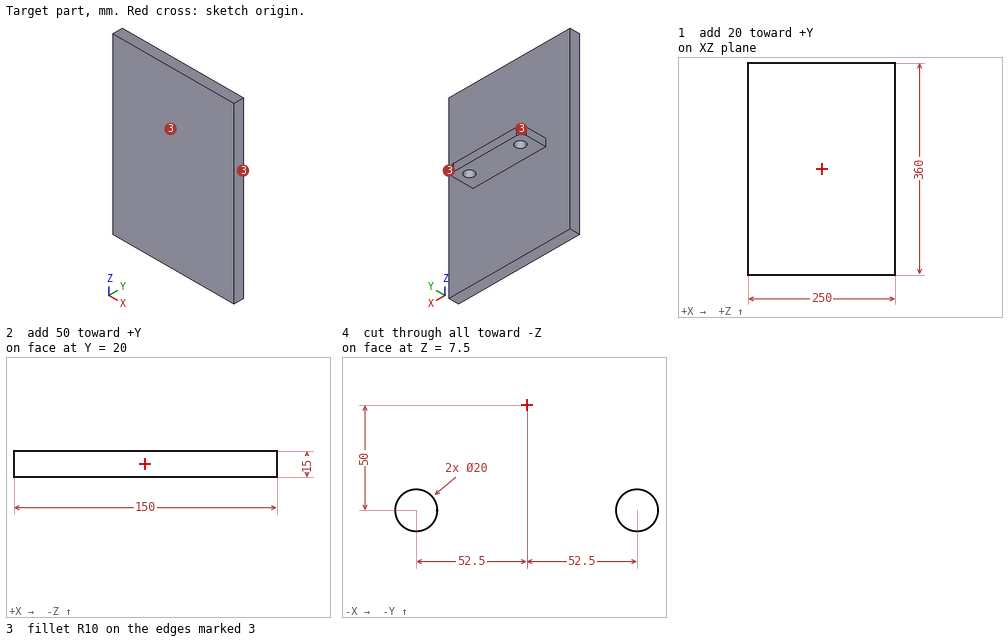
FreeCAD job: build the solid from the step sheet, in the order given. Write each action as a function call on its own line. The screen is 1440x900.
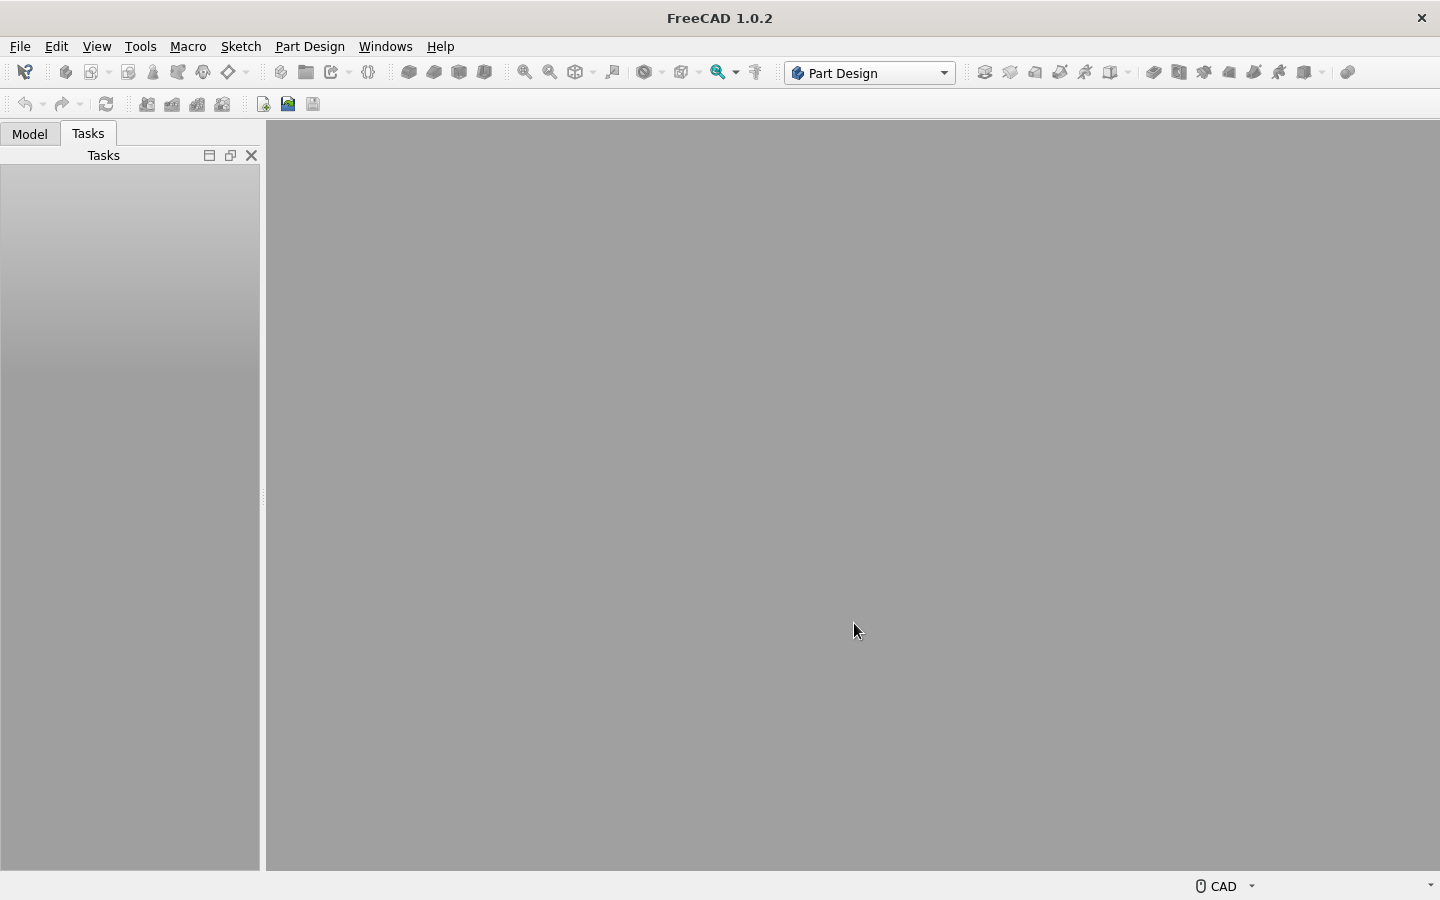
click(263, 104)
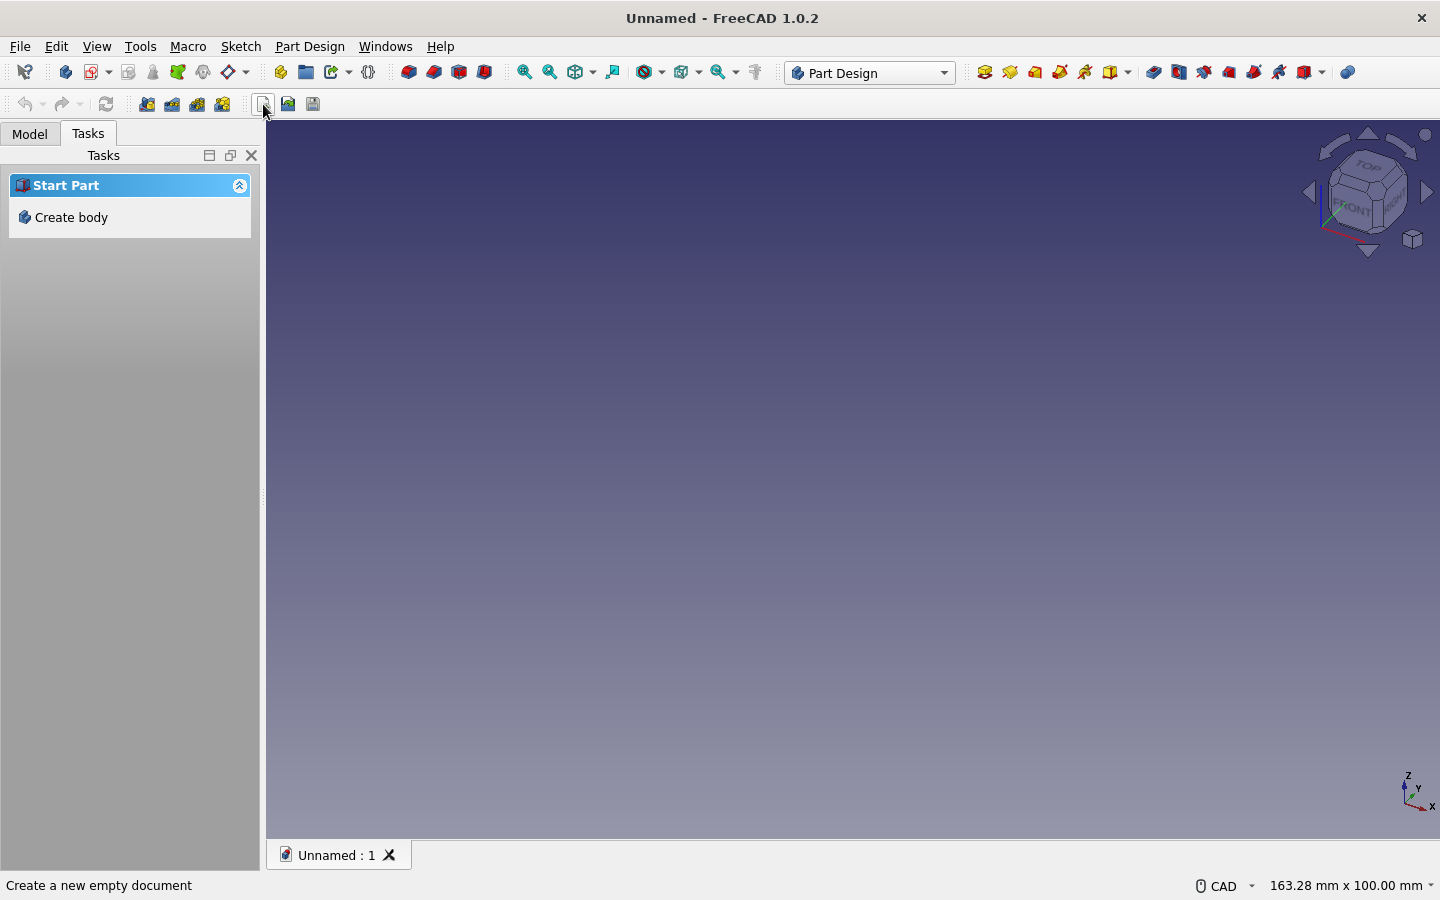
click(90, 72)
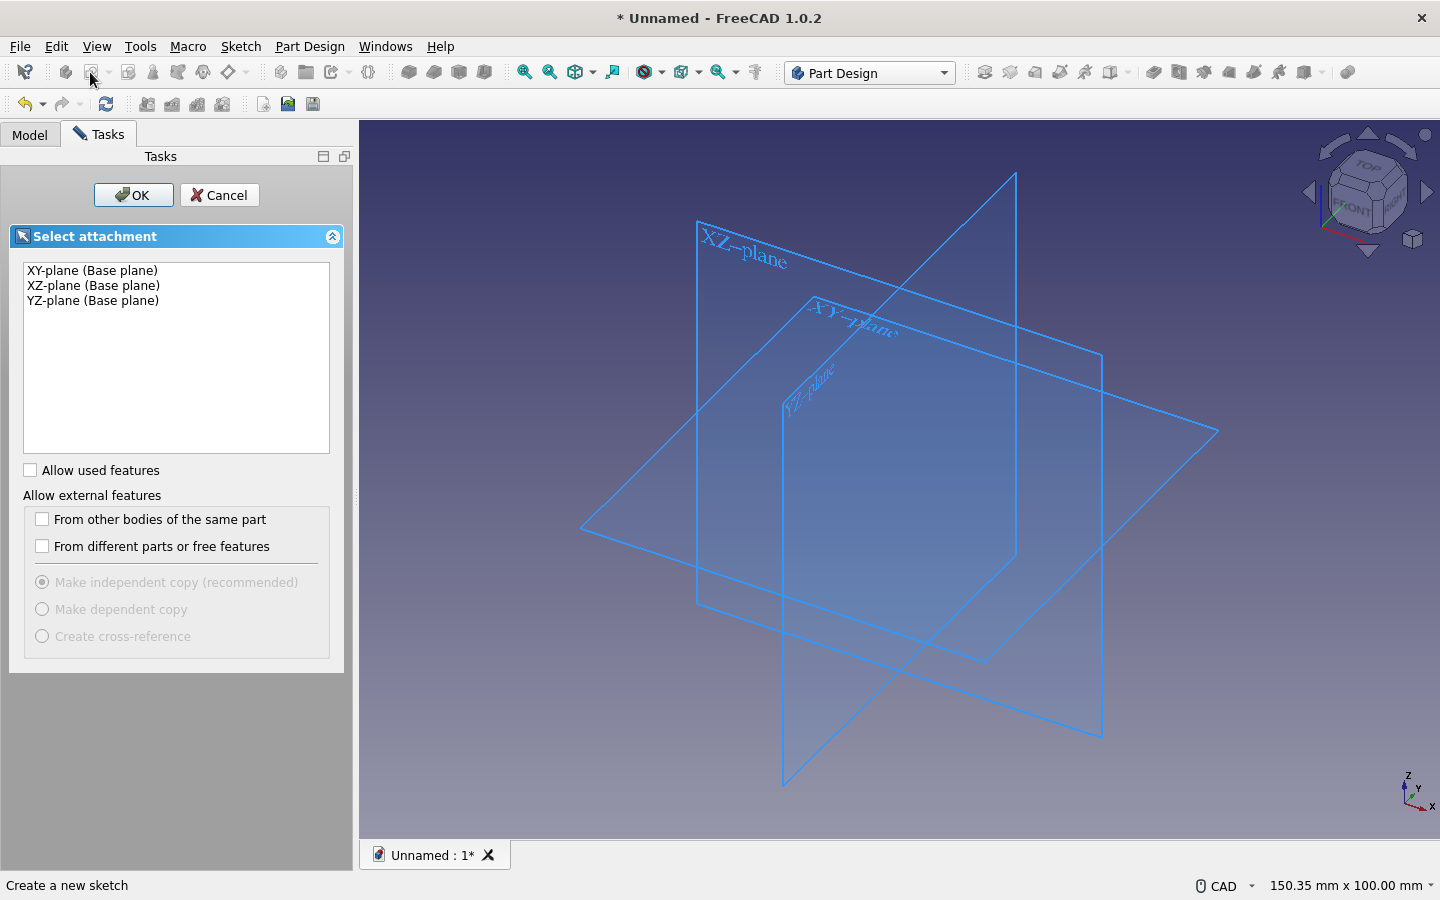
click(84, 286)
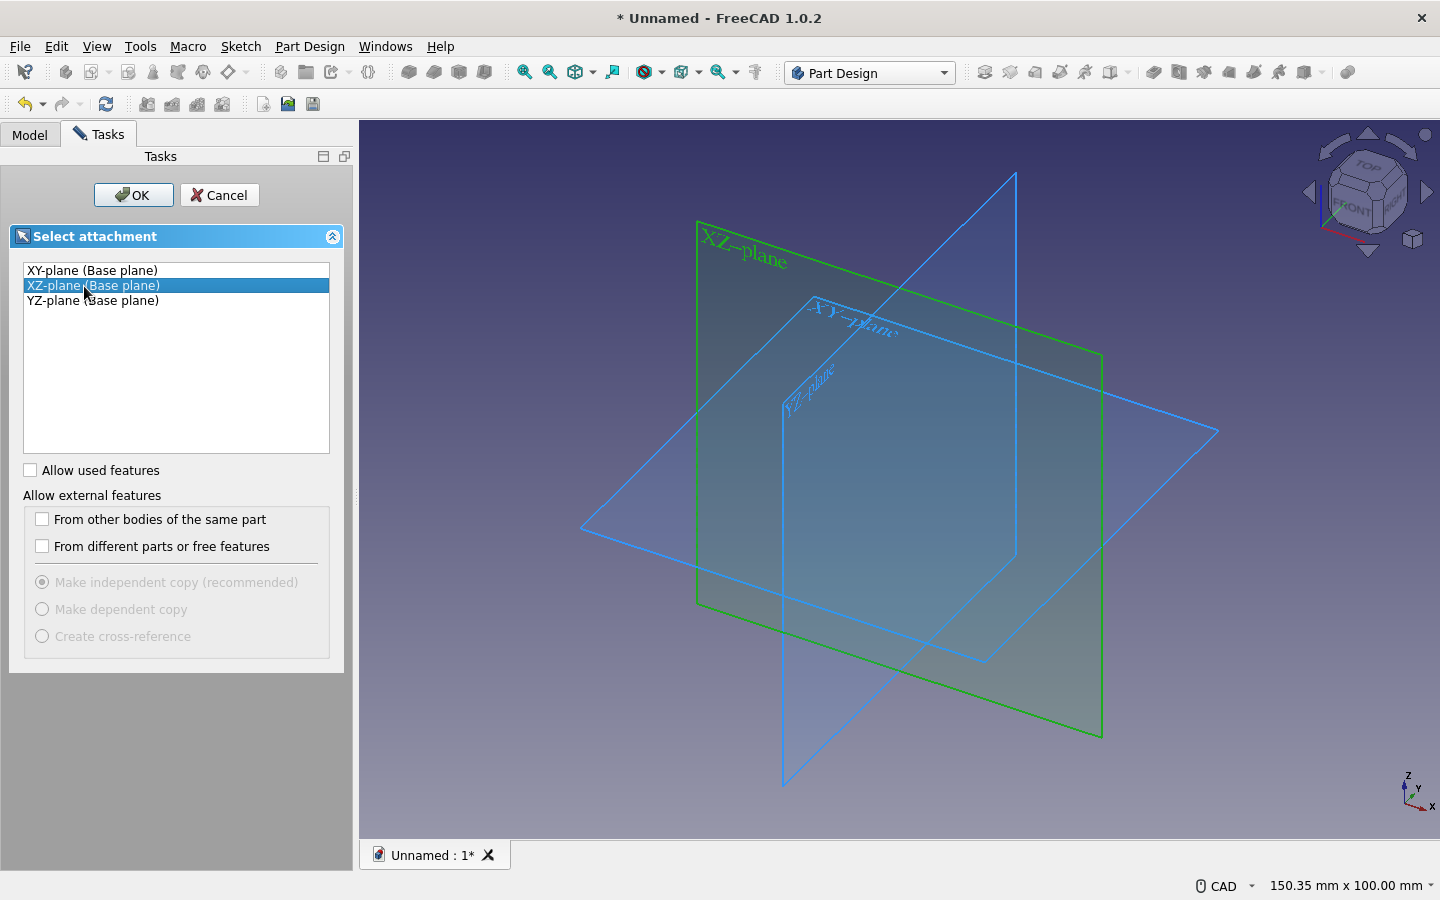
click(134, 195)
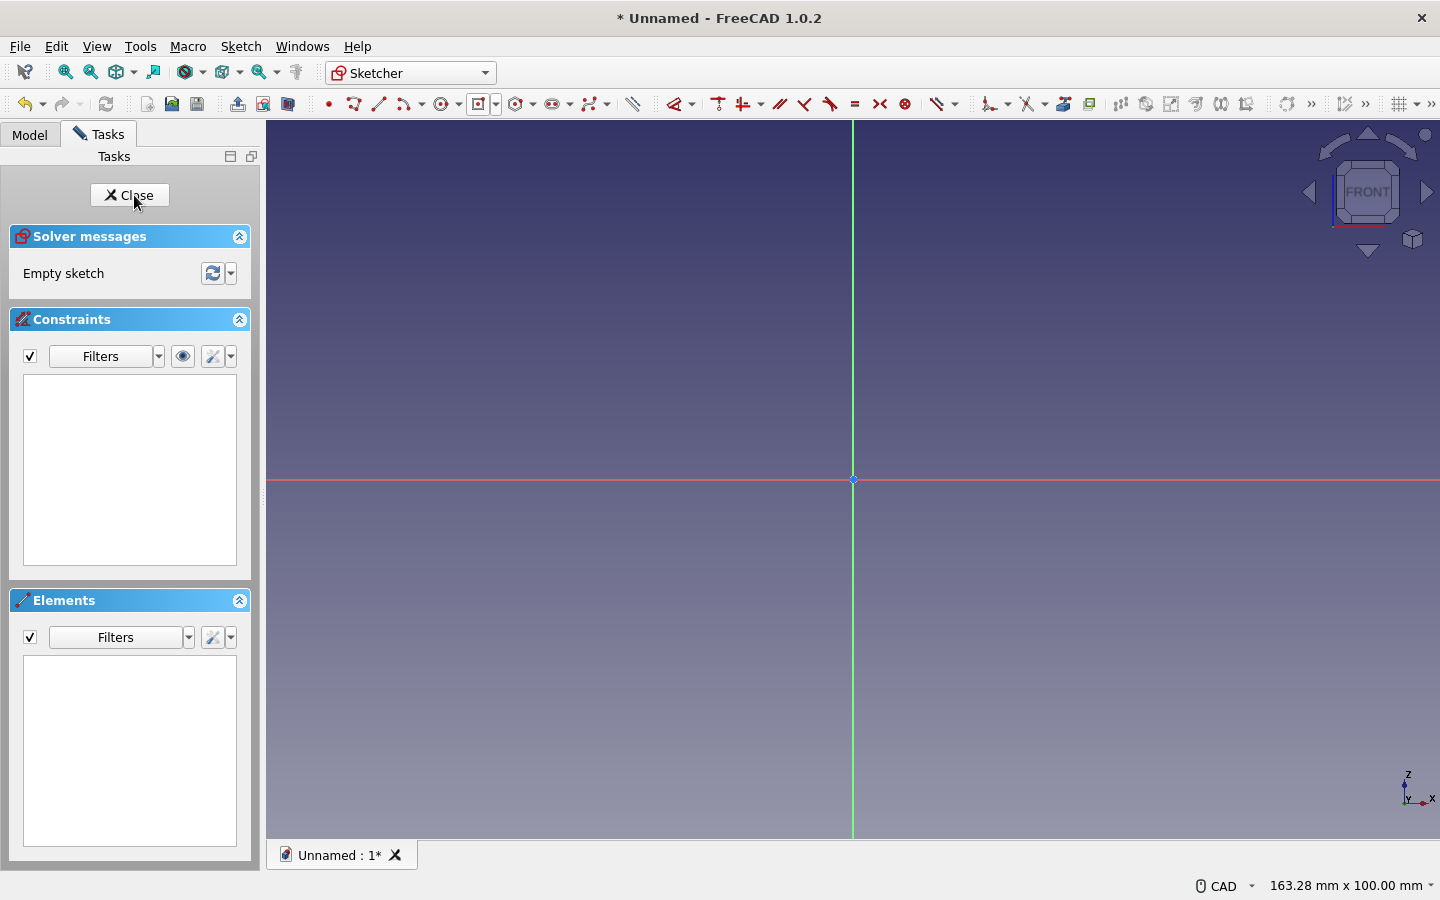
scroll(771, 480, down, 9)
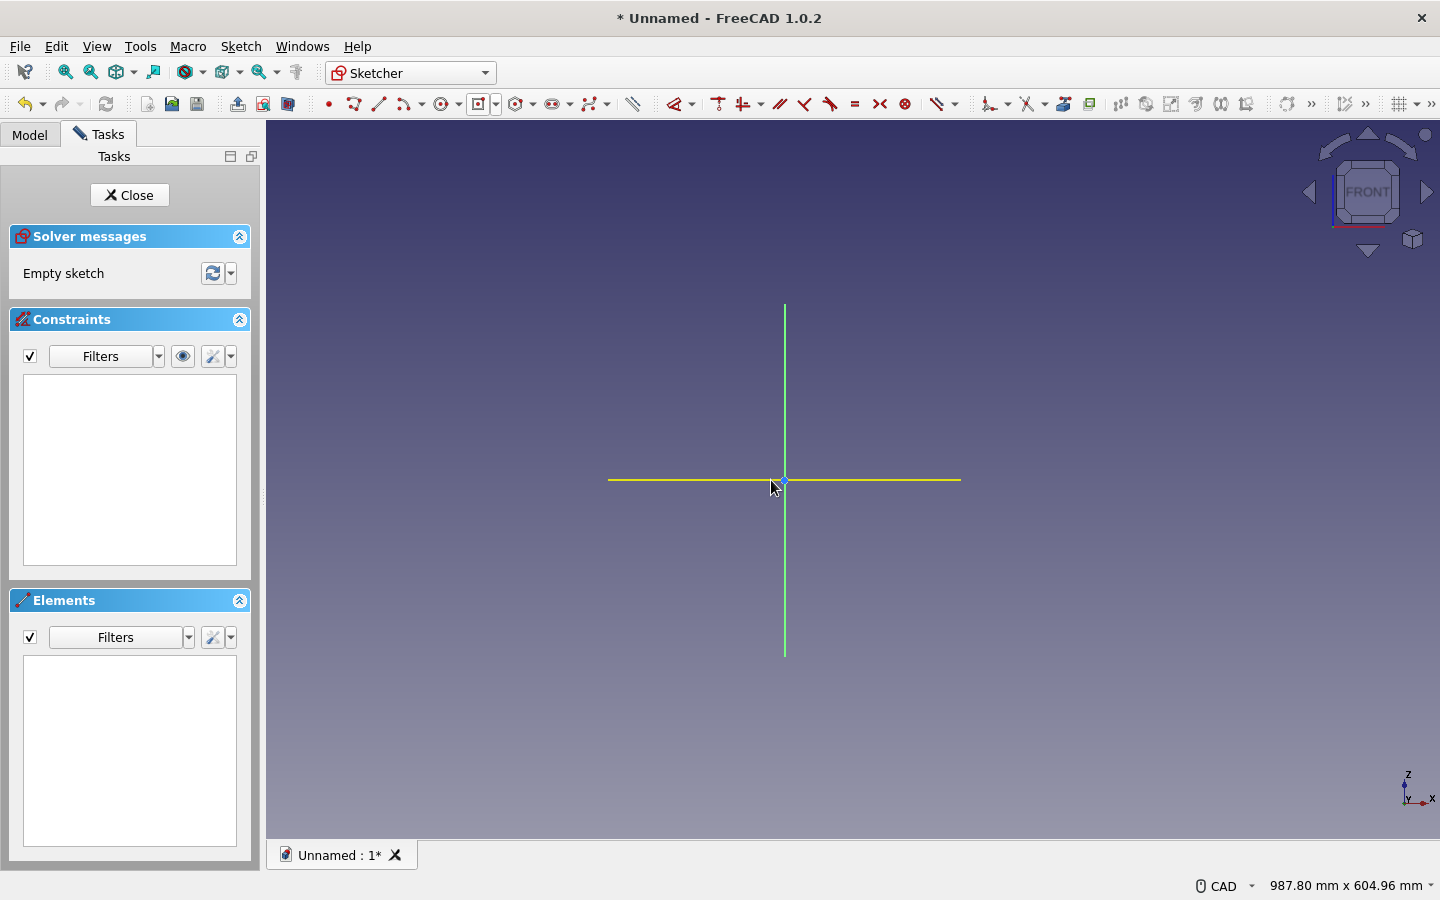
click(478, 104)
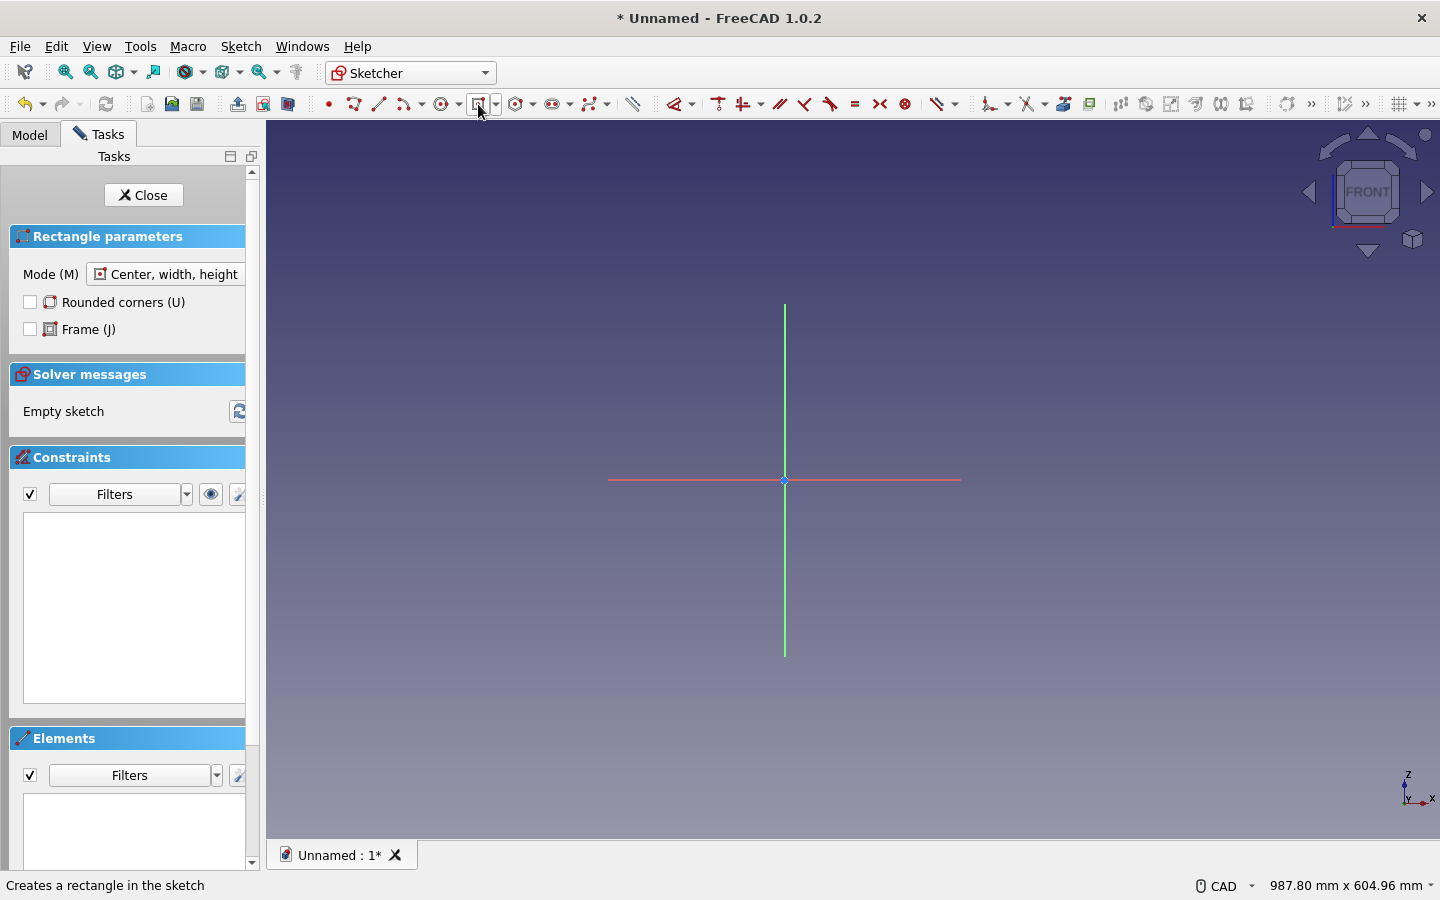
click(785, 480)
click(933, 266)
key(Escape)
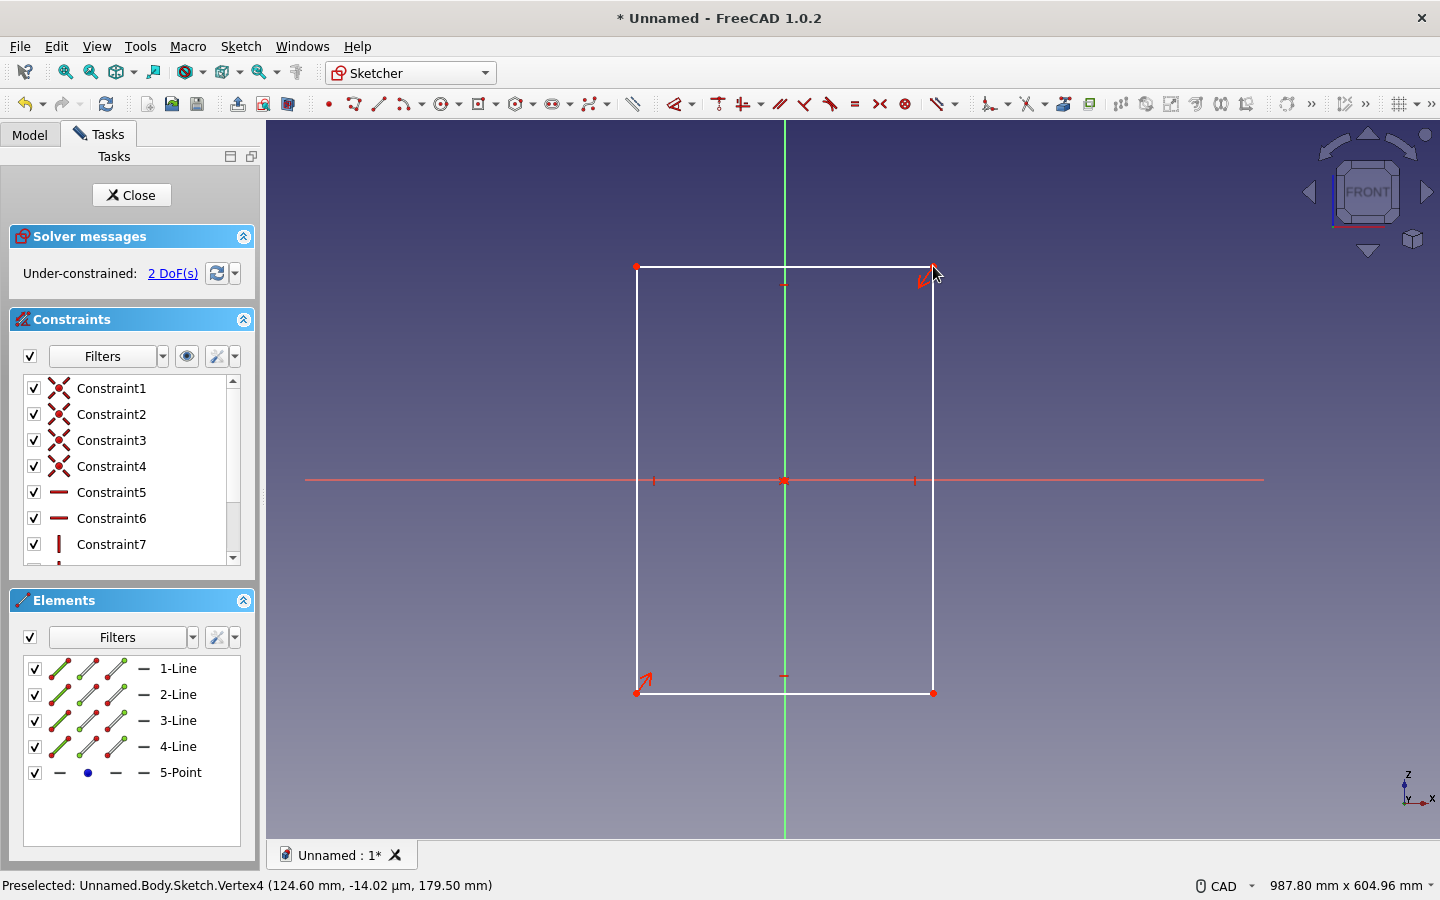
click(674, 104)